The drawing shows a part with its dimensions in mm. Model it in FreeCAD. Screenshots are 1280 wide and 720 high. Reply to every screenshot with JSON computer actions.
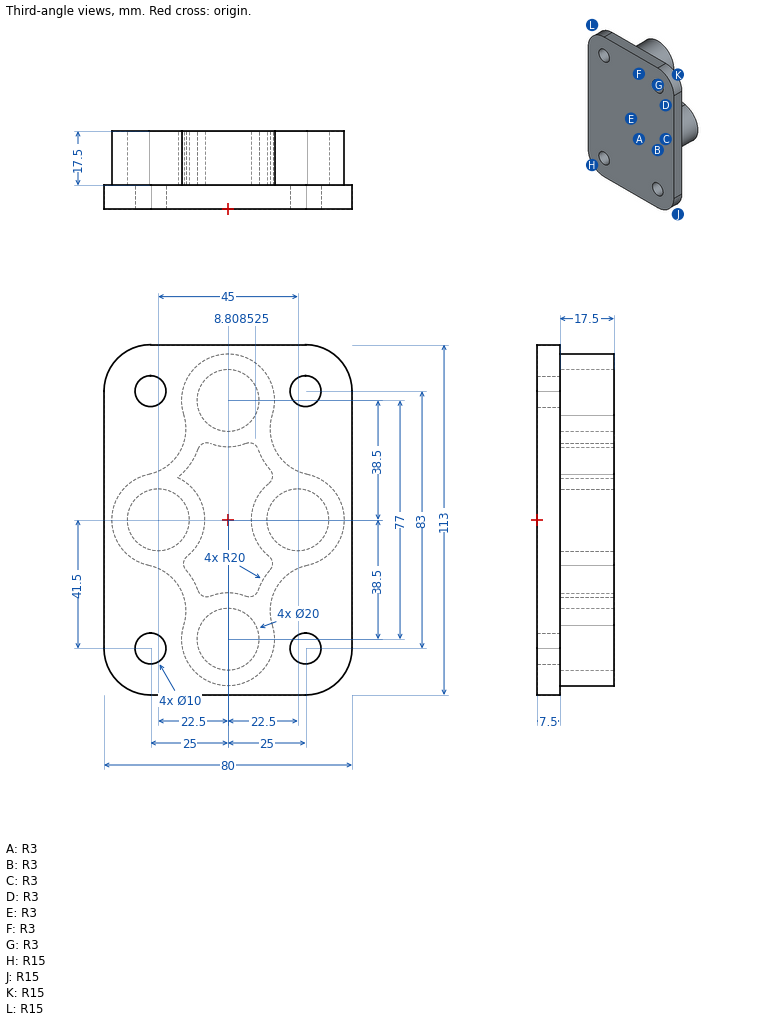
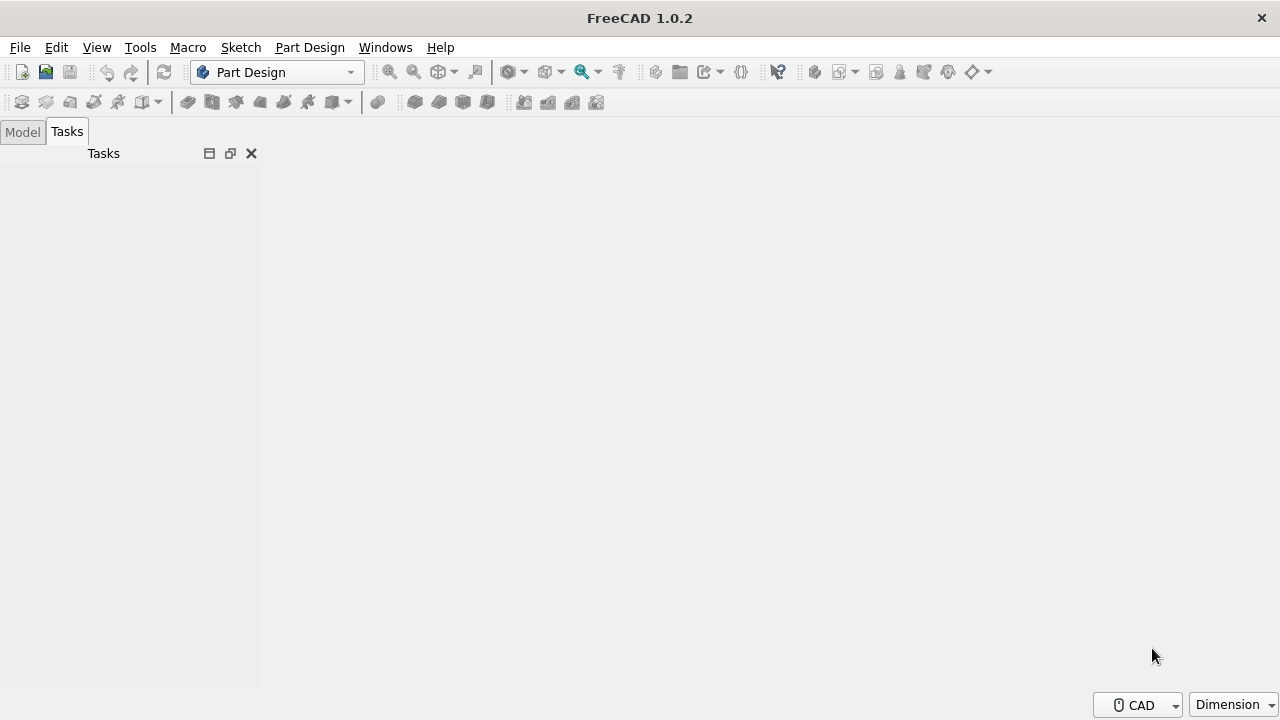
{"action": "key", "text": "ctrl+n"}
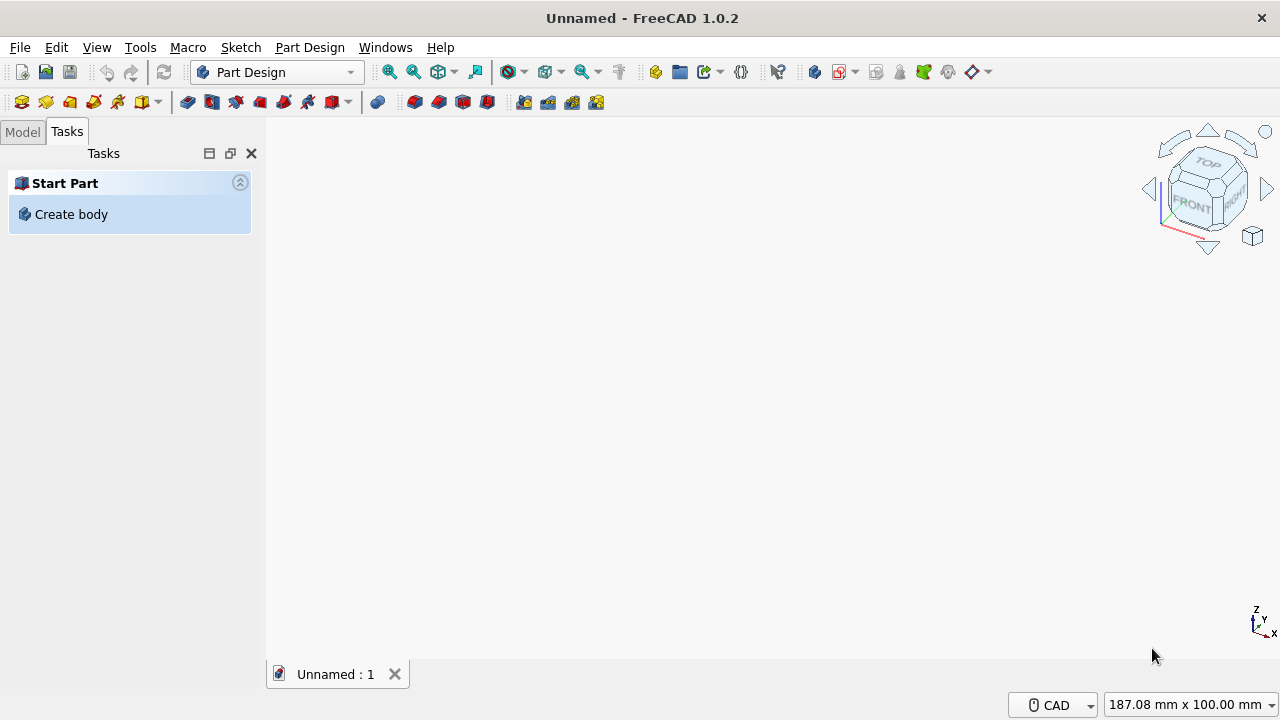
{"action": "left_click", "coordinate": [840, 72]}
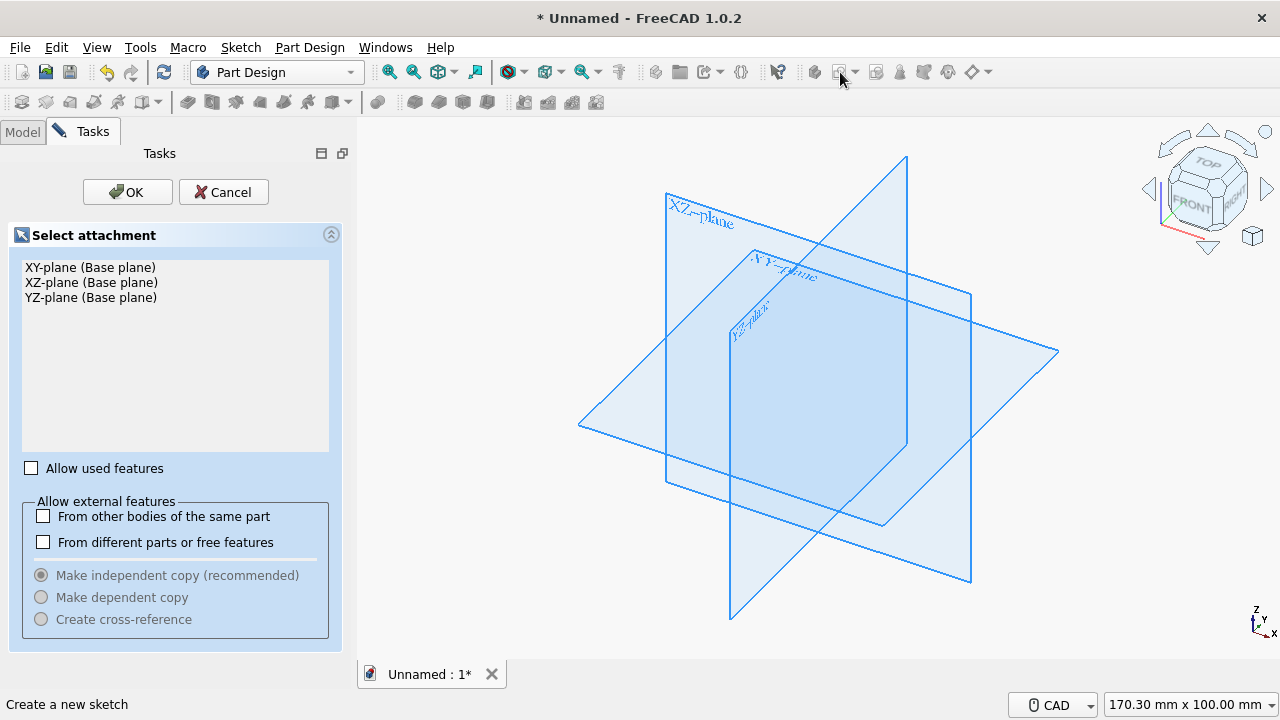
{"action": "left_click", "coordinate": [82, 282]}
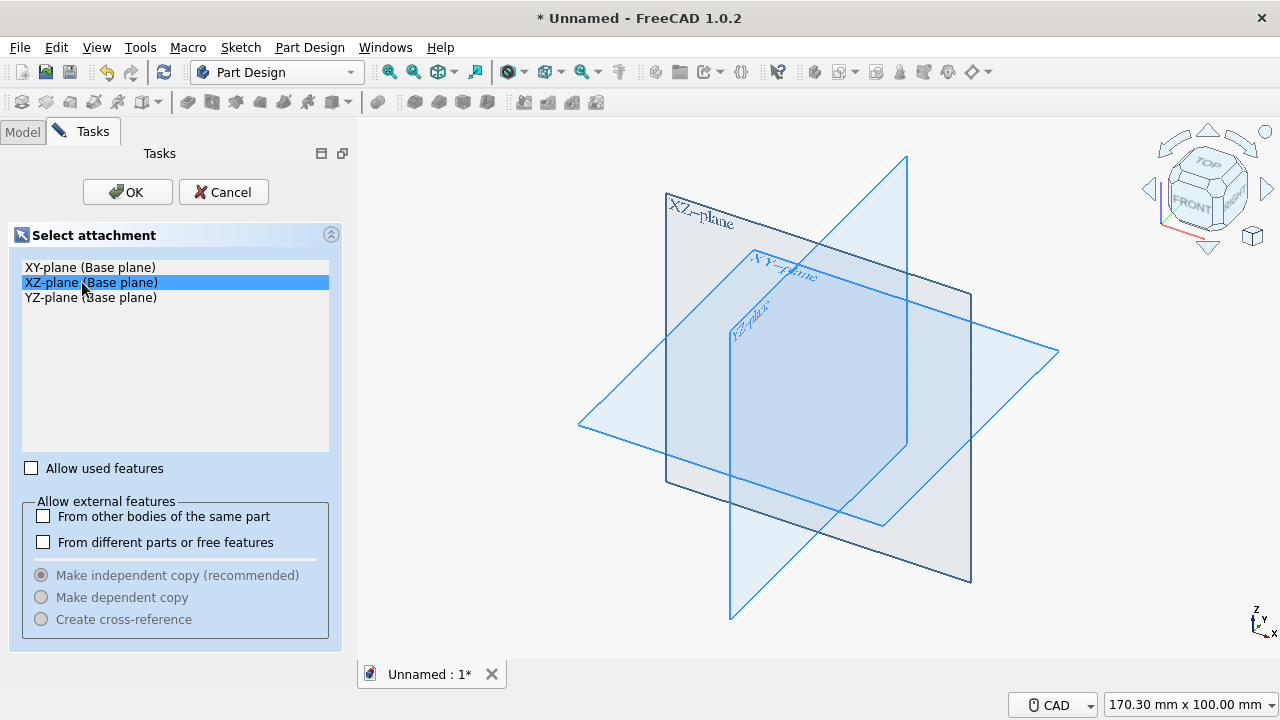
{"action": "left_click", "coordinate": [128, 192]}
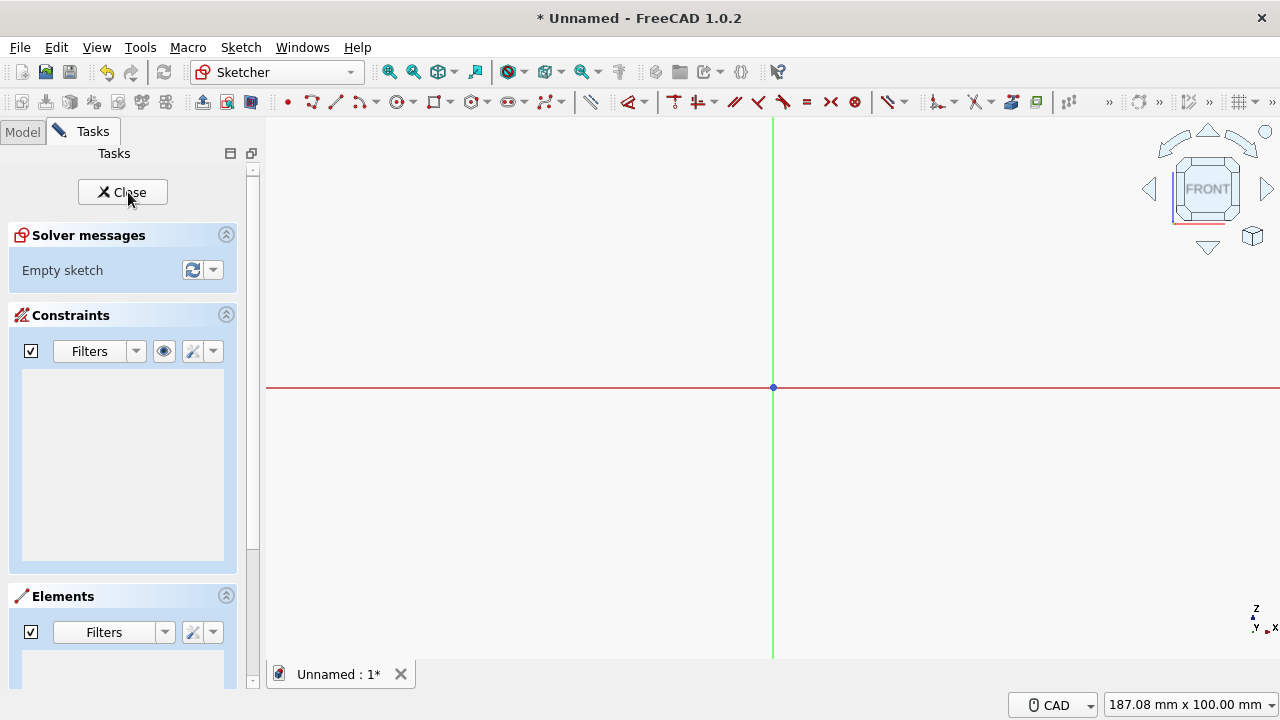
{"action": "scroll", "coordinate": [621, 388], "scroll_direction": "down", "scroll_amount": 3}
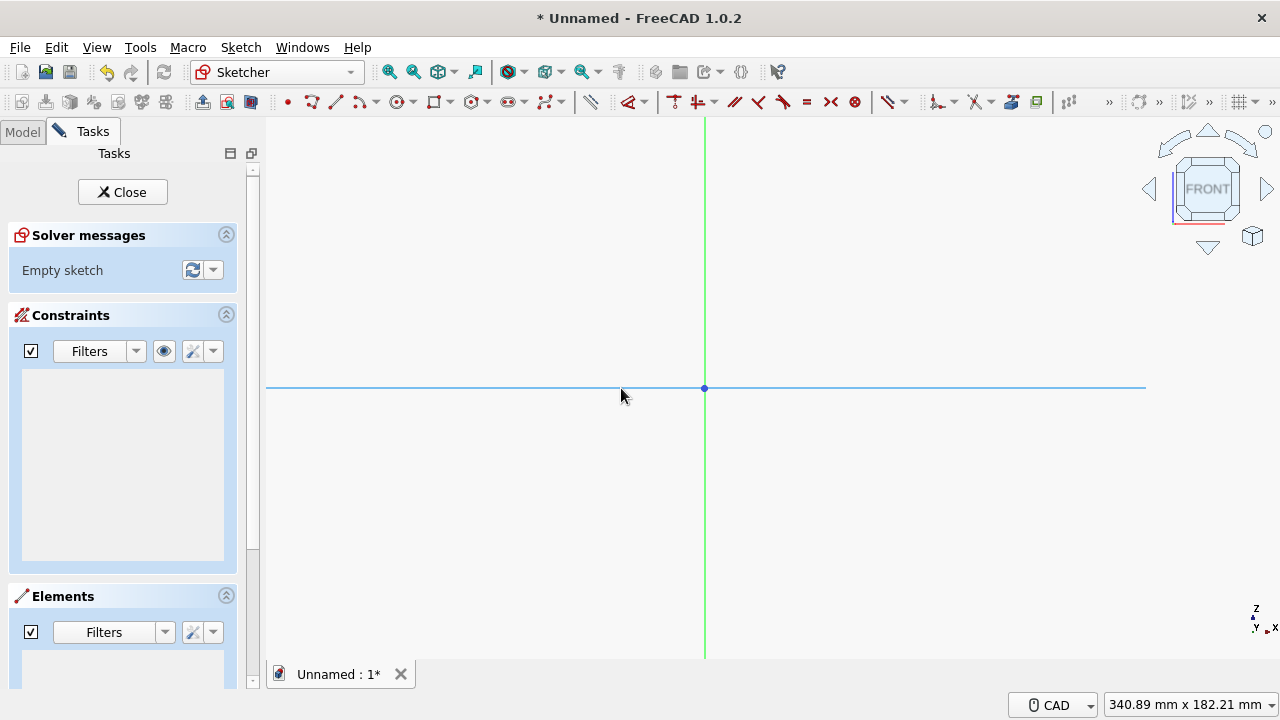
{"action": "key", "text": "g v"}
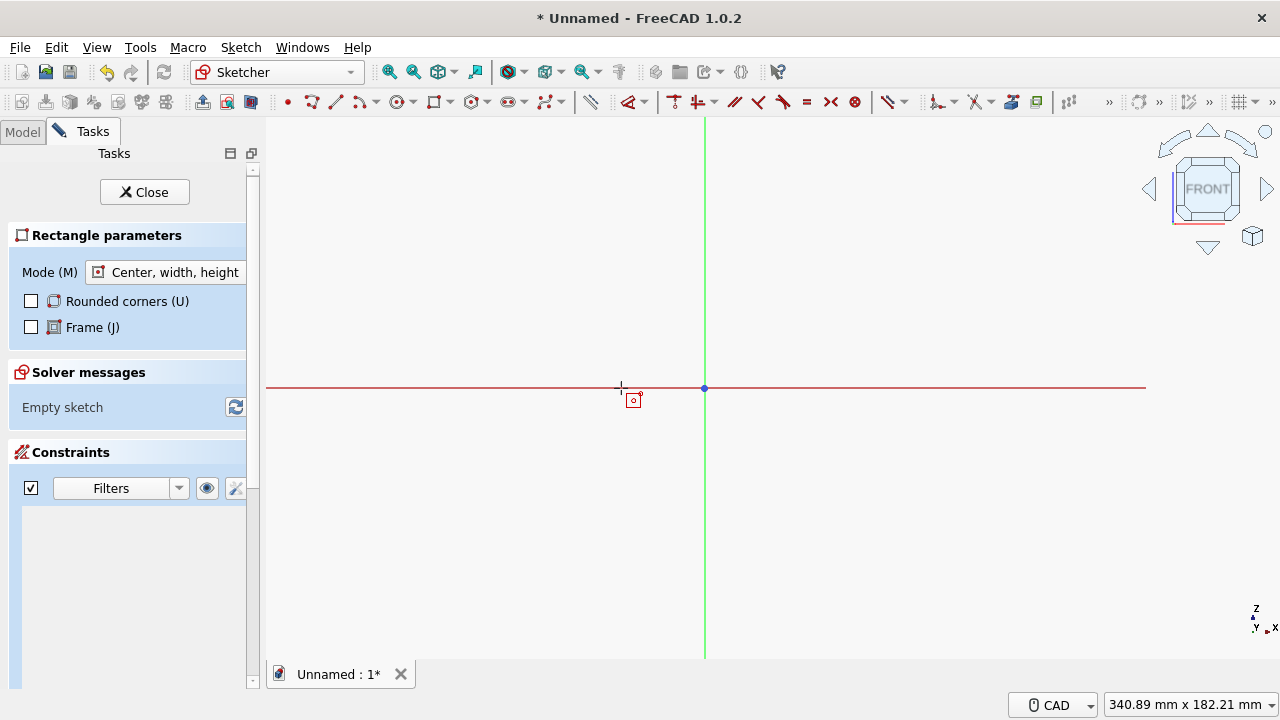
{"action": "left_click", "coordinate": [705, 388]}
{"action": "mouse_move", "coordinate": [824, 220]}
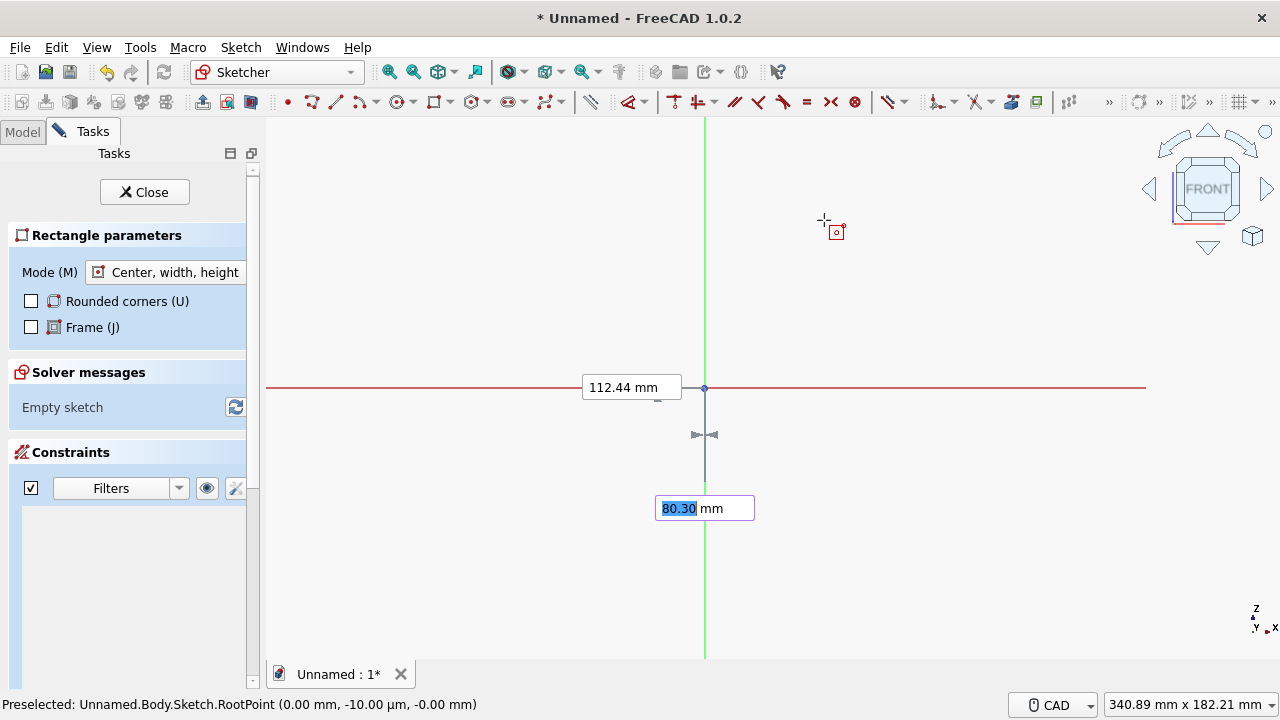
{"action": "type", "text": "80"}
{"action": "key", "text": "Tab"}
{"action": "type", "text": "113"}
{"action": "key", "text": "Return"}
{"action": "key", "text": "Escape"}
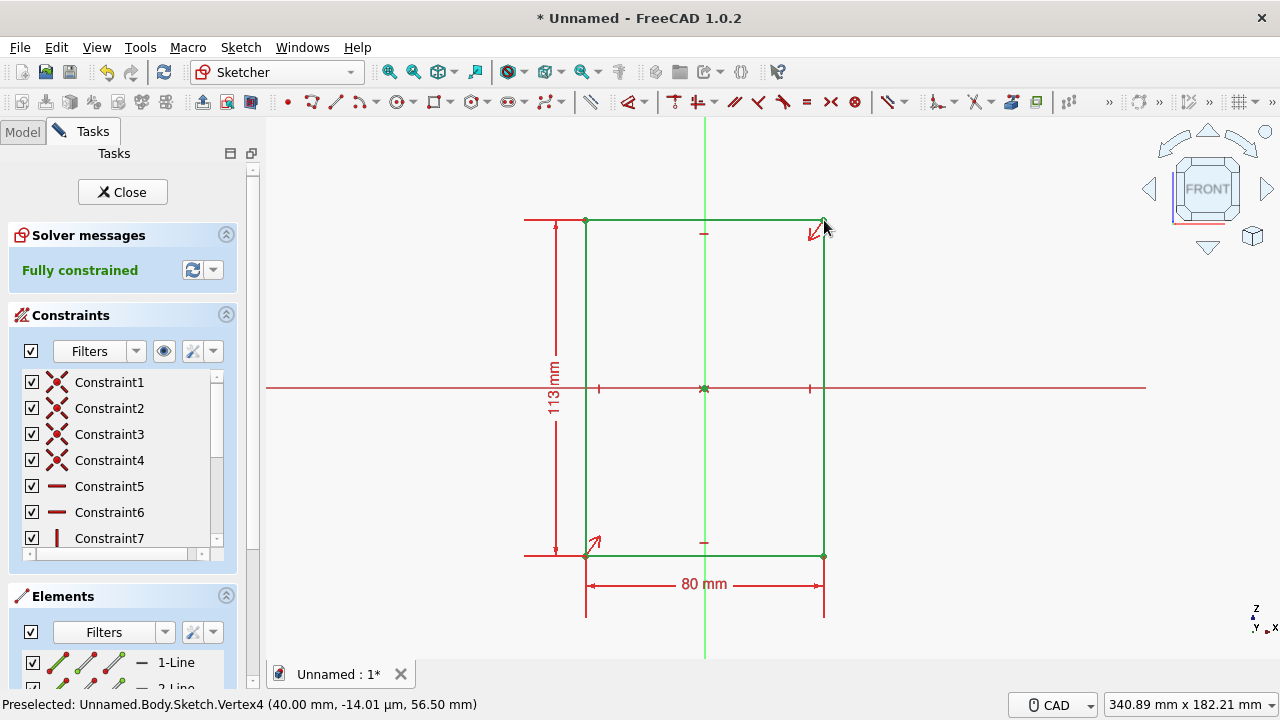
{"action": "left_click", "coordinate": [123, 192]}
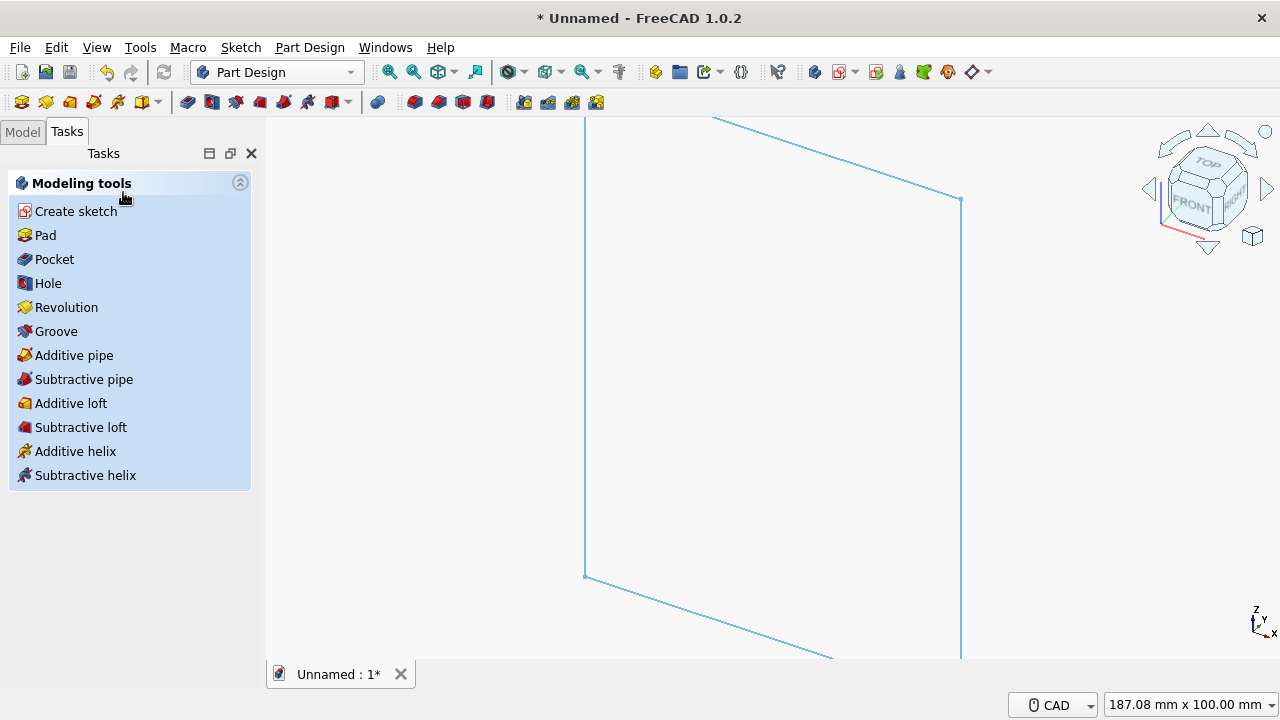
{"action": "left_click", "coordinate": [22, 102]}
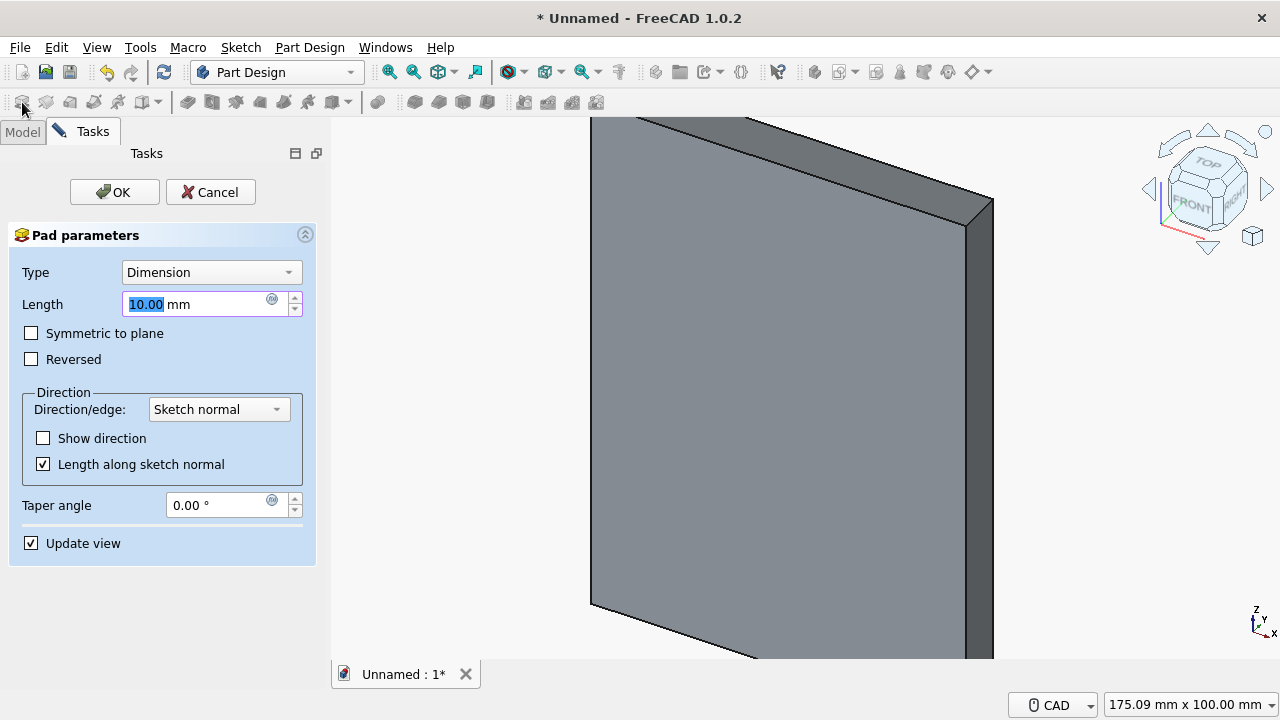
{"action": "type", "text": "7.5"}
{"action": "key", "text": "Tab"}